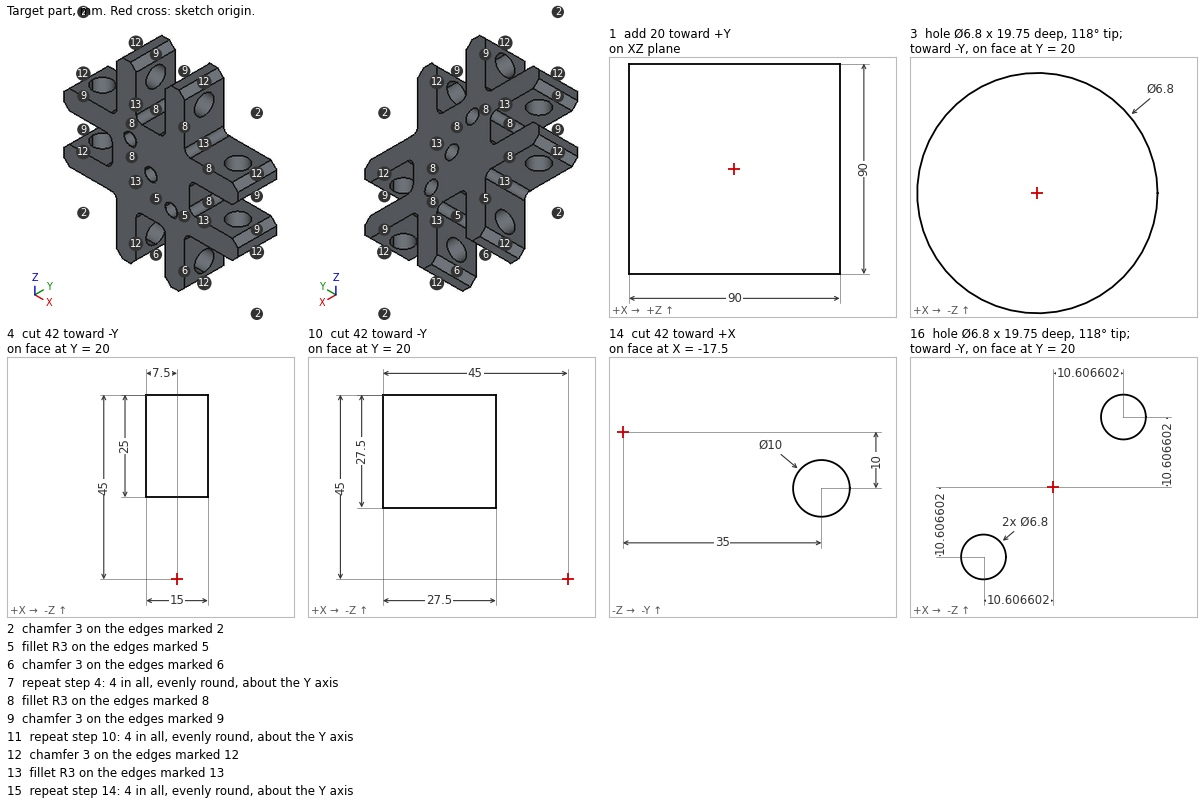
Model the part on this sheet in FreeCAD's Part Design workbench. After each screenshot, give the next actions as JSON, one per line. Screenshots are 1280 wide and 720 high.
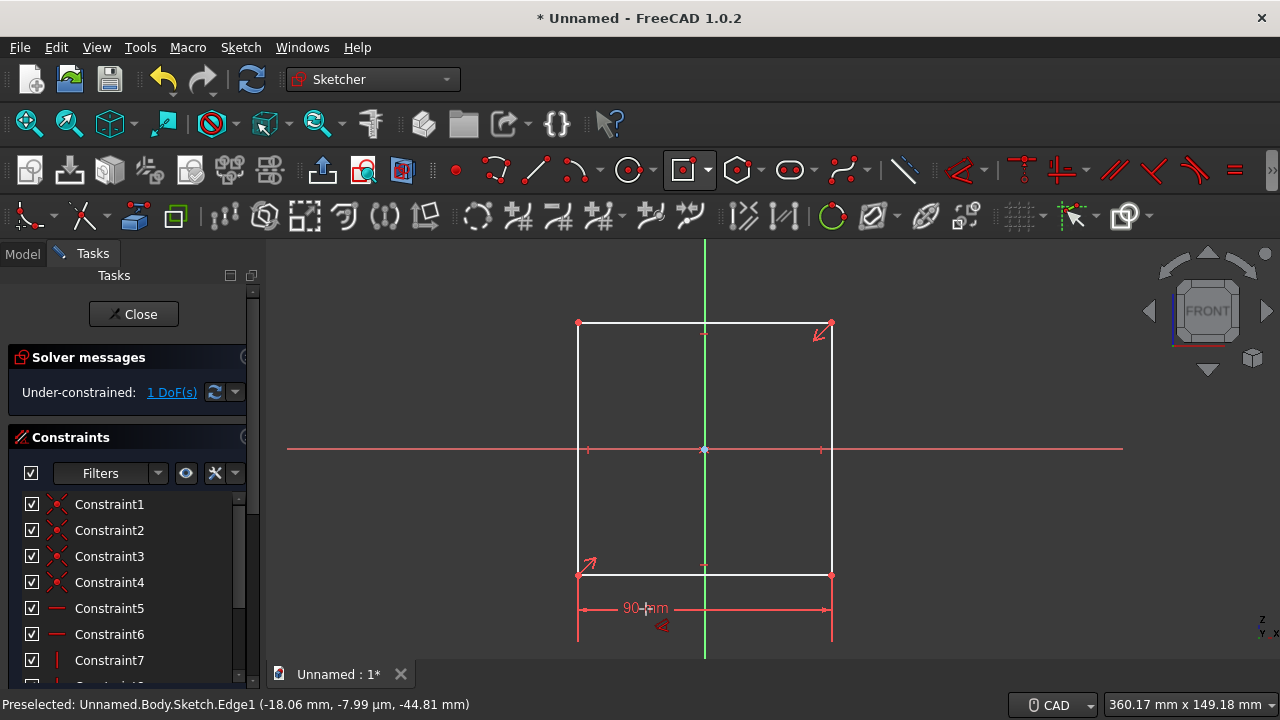
{"action": "left_click", "coordinate": [832, 500]}
{"action": "left_click", "coordinate": [866, 391]}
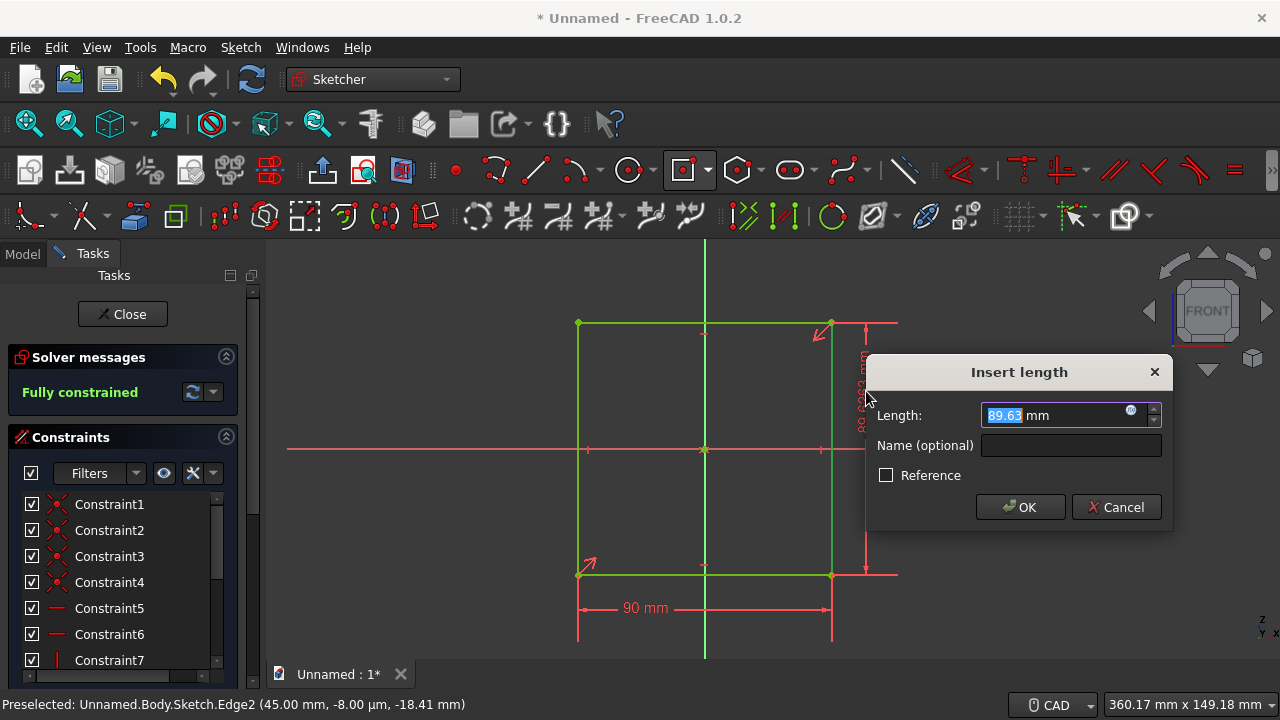
{"action": "type", "text": "90"}
{"action": "key", "text": "Return"}
{"action": "key", "text": "Escape"}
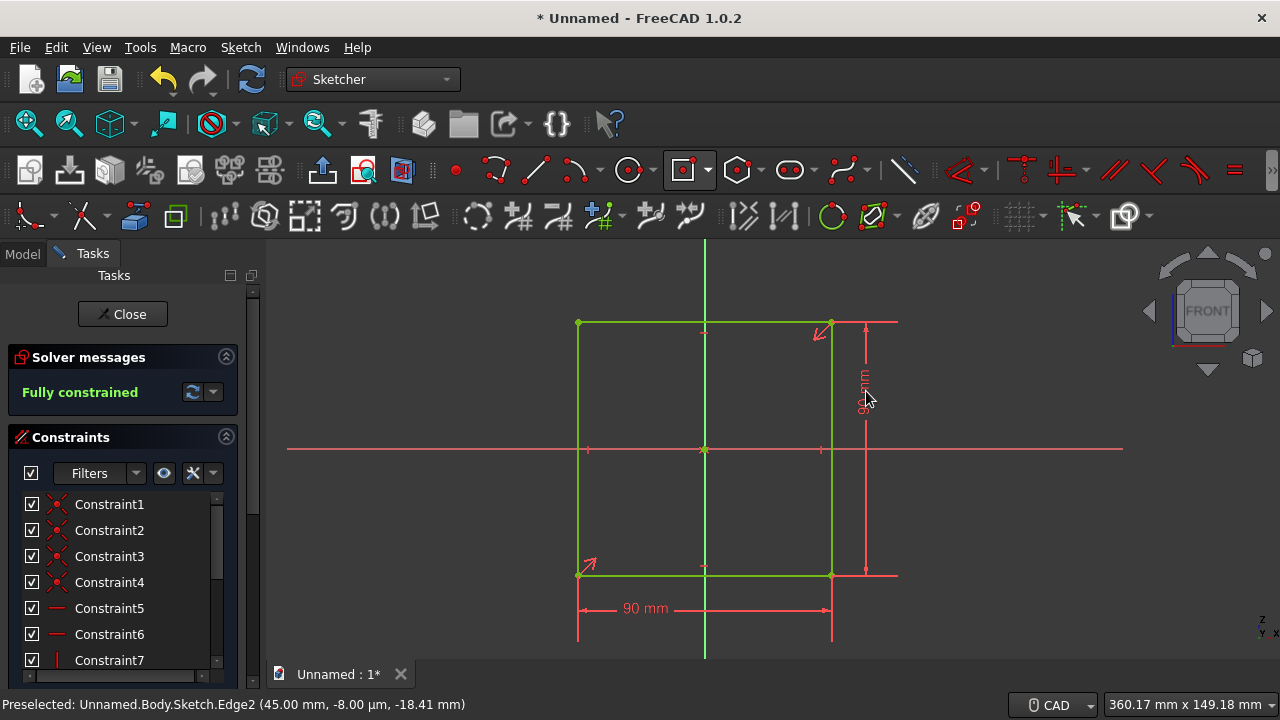
{"action": "left_click", "coordinate": [123, 314]}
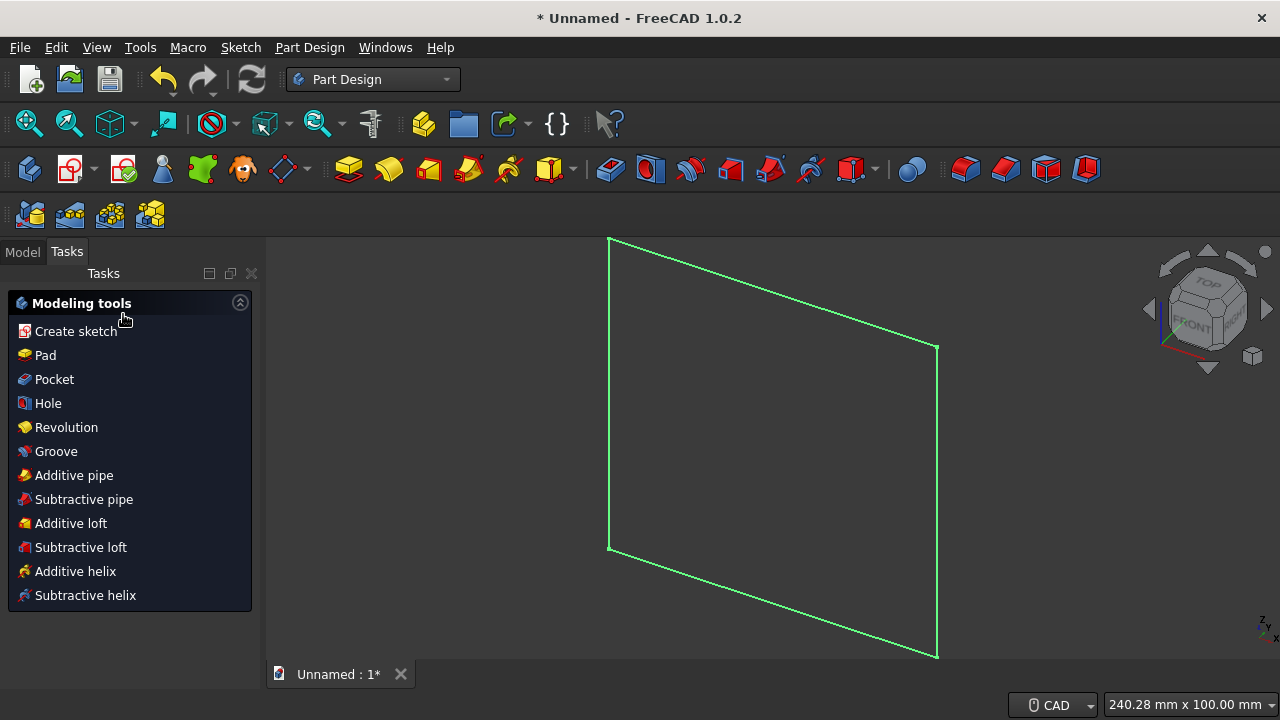
{"action": "left_click", "coordinate": [350, 170]}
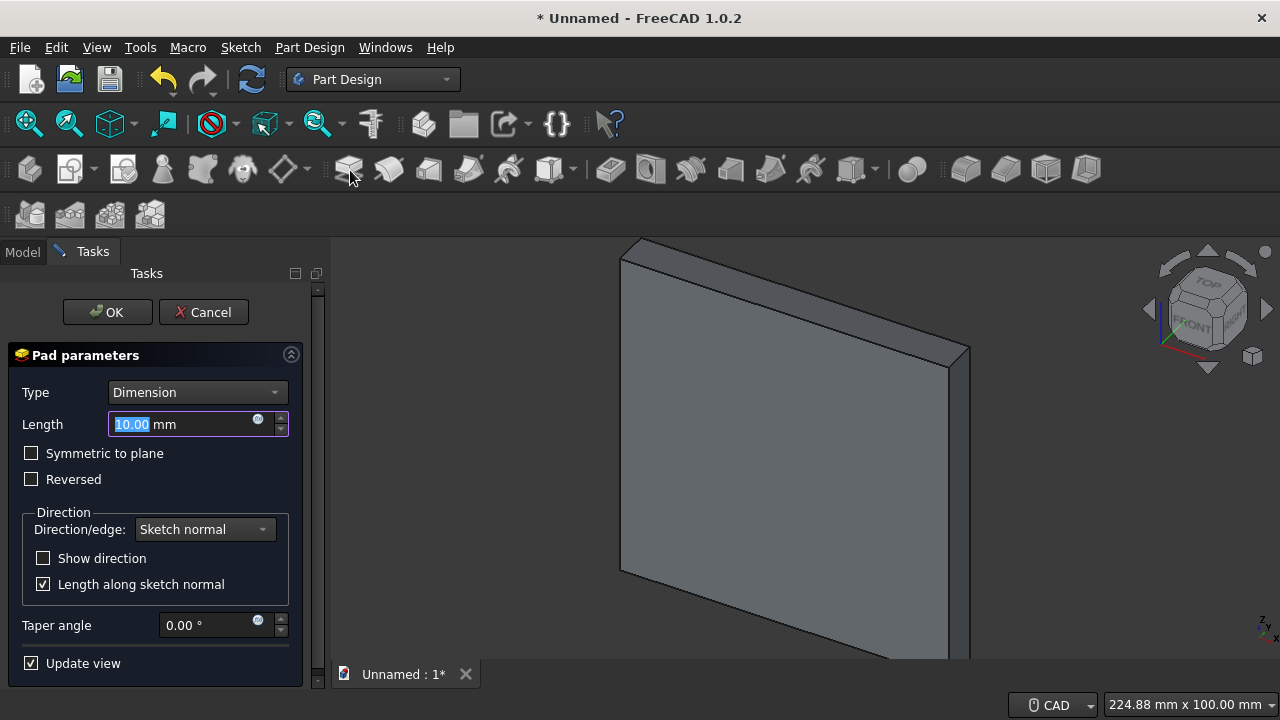
{"action": "type", "text": "20"}
{"action": "key", "text": "Tab"}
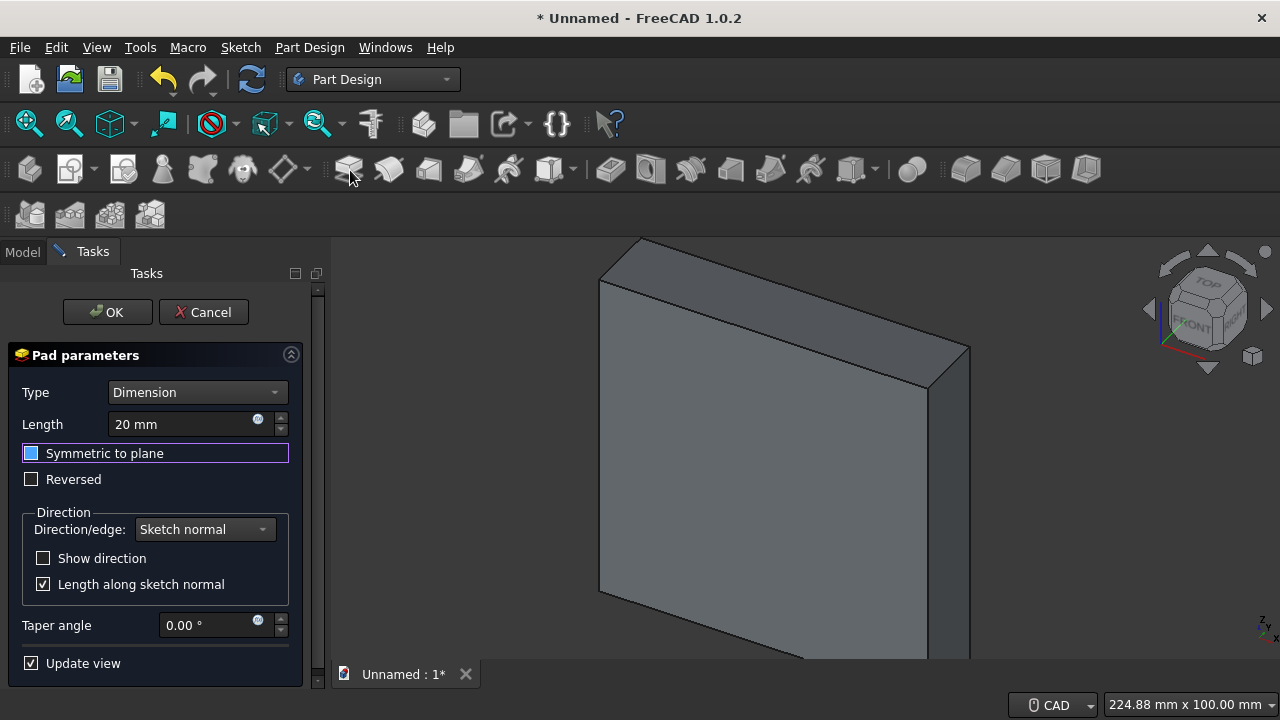
{"action": "left_click", "coordinate": [30, 479]}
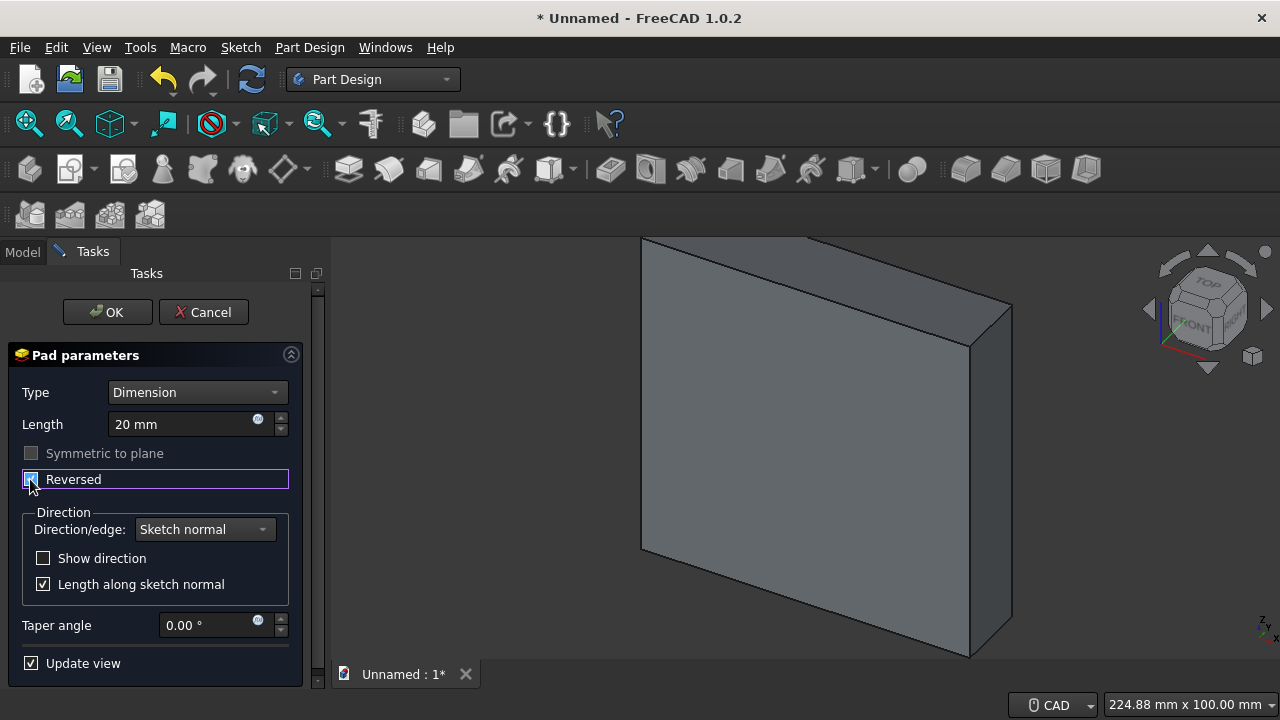
{"action": "left_click", "coordinate": [108, 312]}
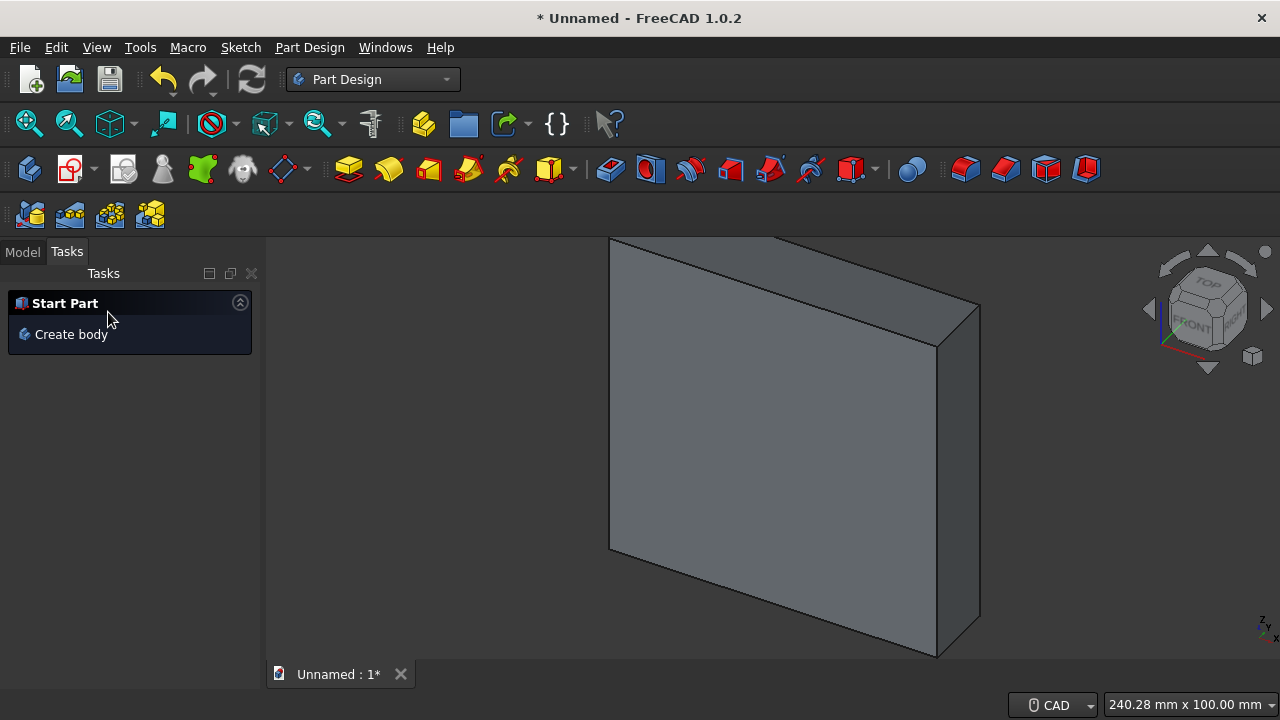
{"action": "left_click", "coordinate": [30, 124]}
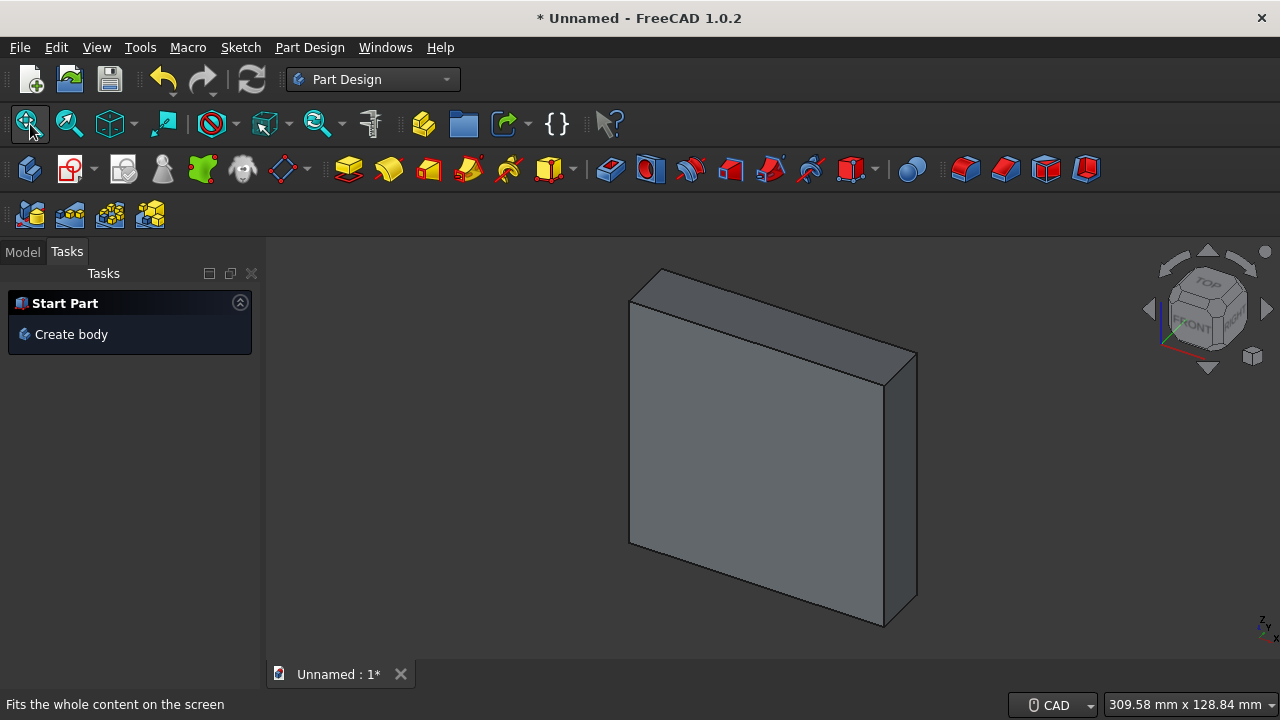
{"action": "left_click", "coordinate": [901, 369]}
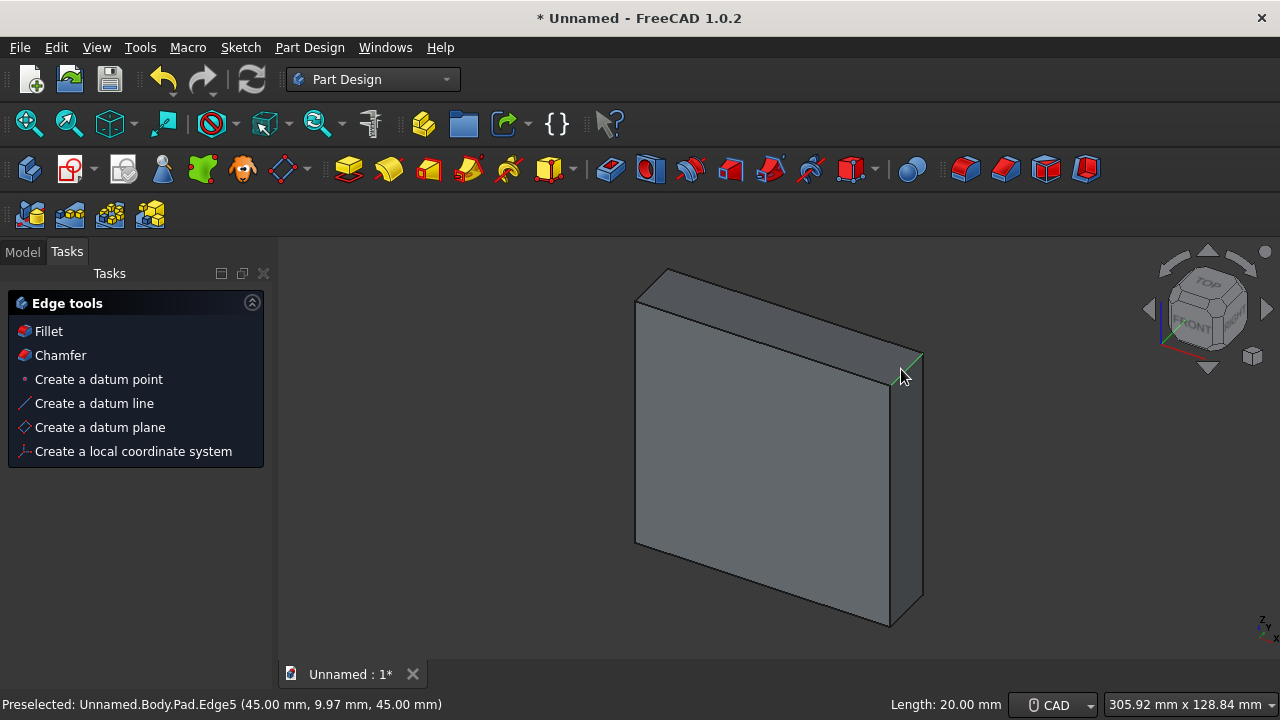
{"action": "key", "text": "0"}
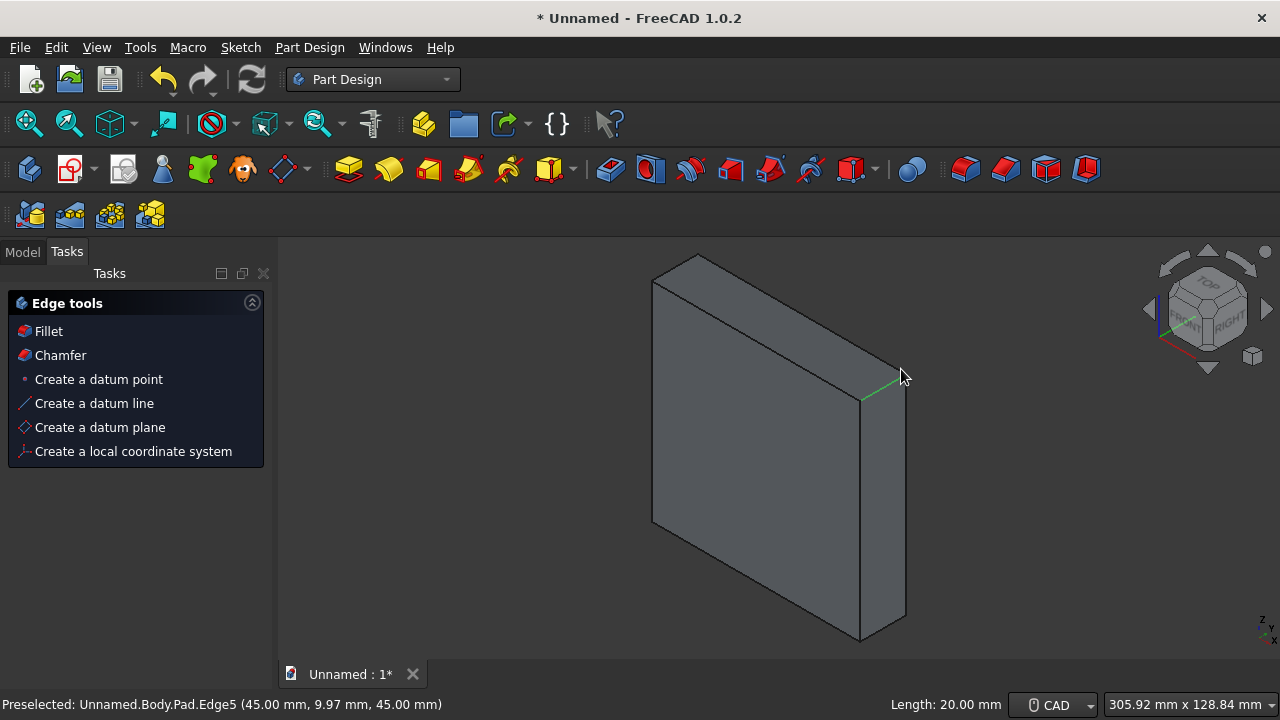
{"action": "key", "text": "2"}